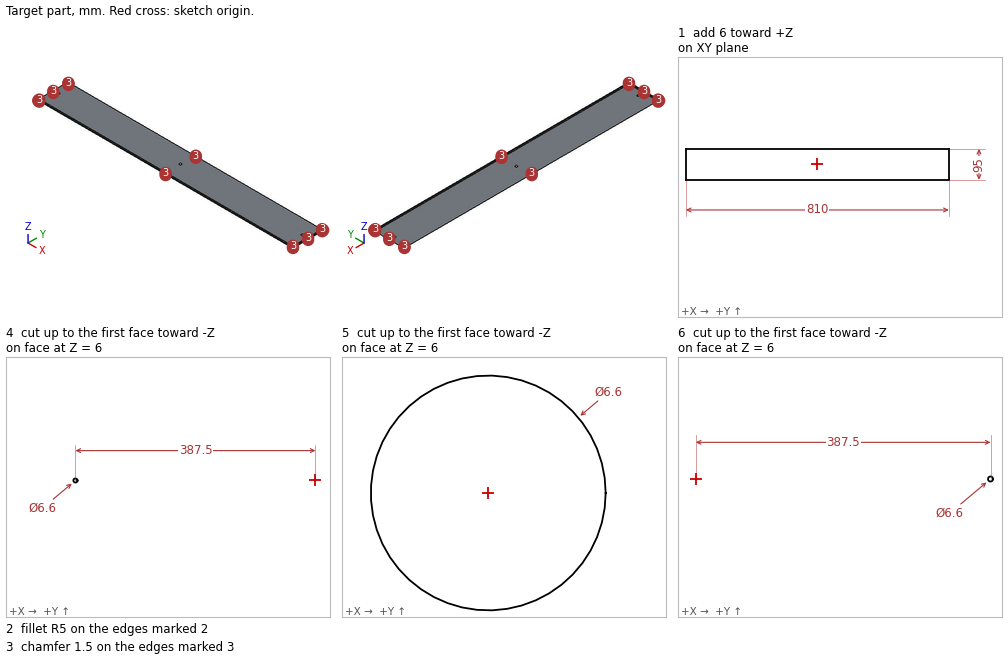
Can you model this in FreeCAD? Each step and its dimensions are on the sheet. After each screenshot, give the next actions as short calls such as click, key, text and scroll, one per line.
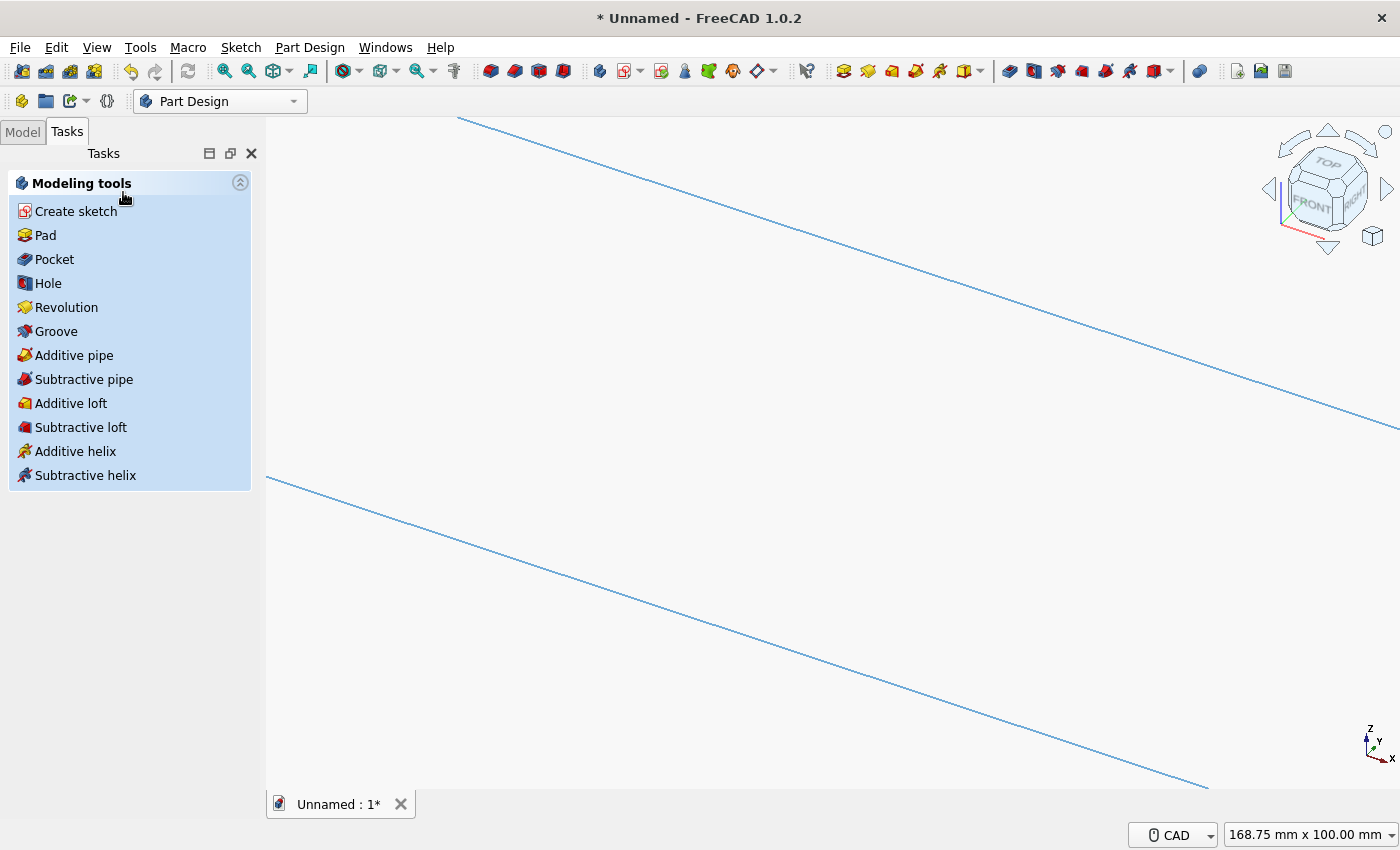
click(844, 72)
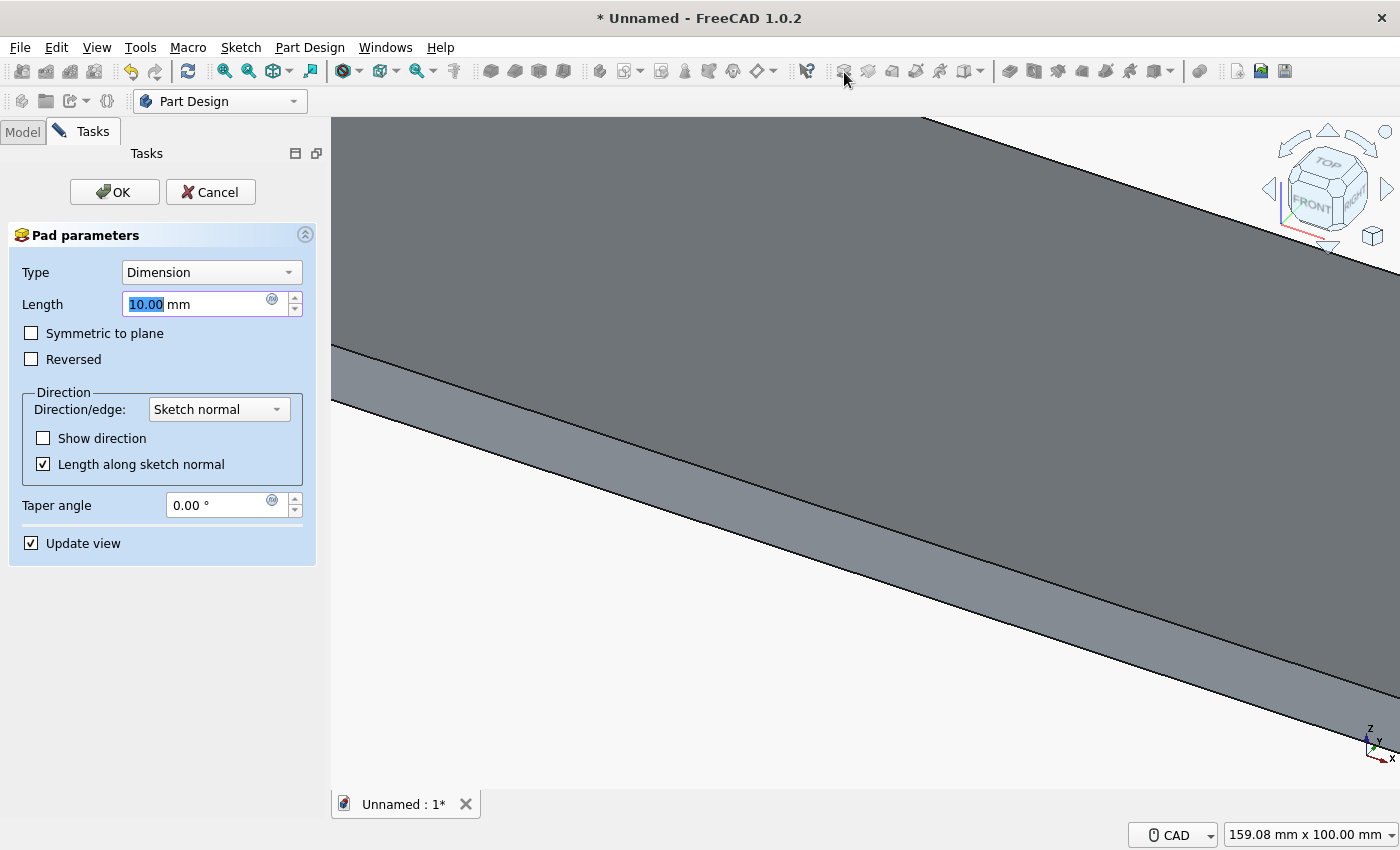
text(6)
key(Tab)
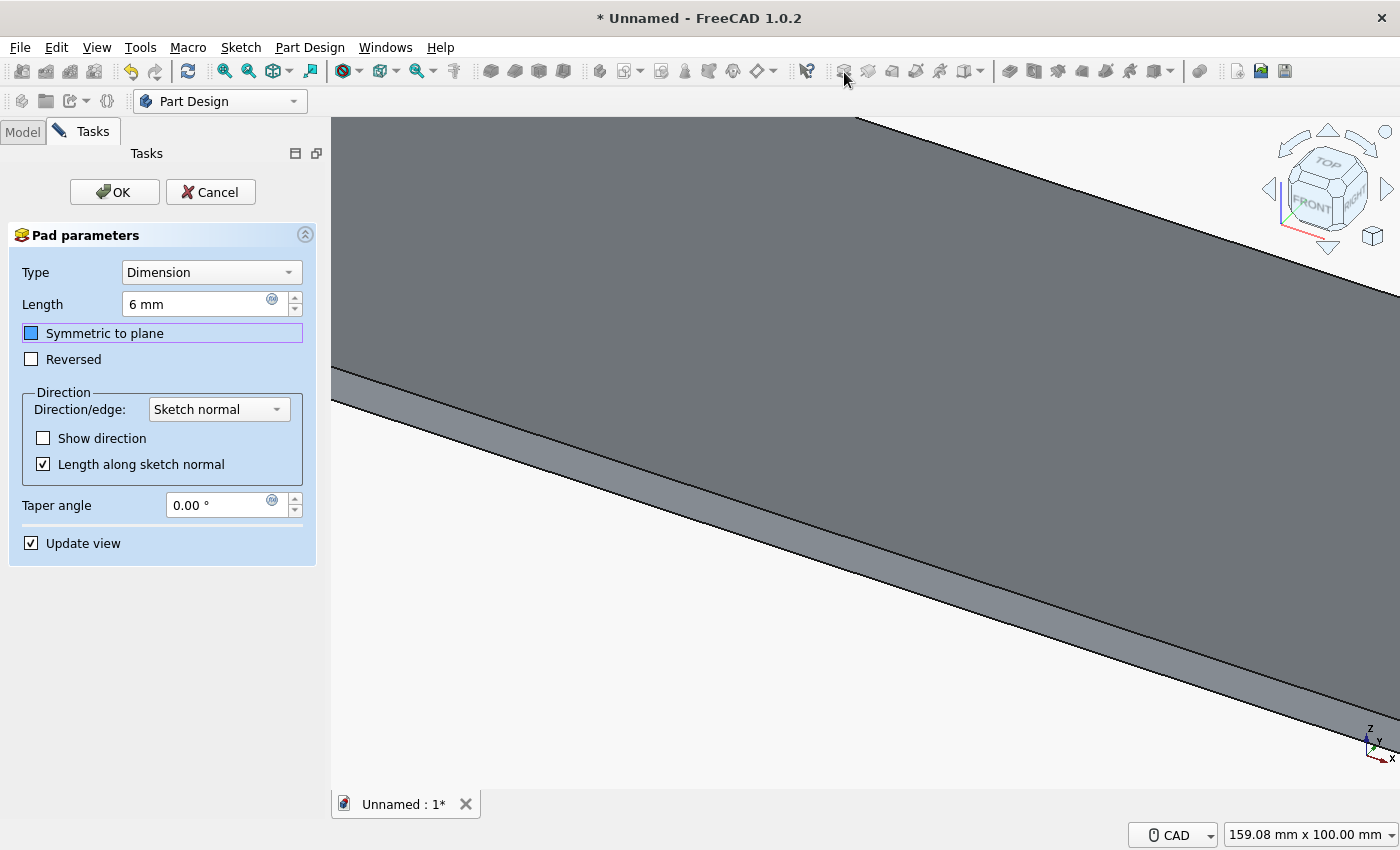
click(115, 192)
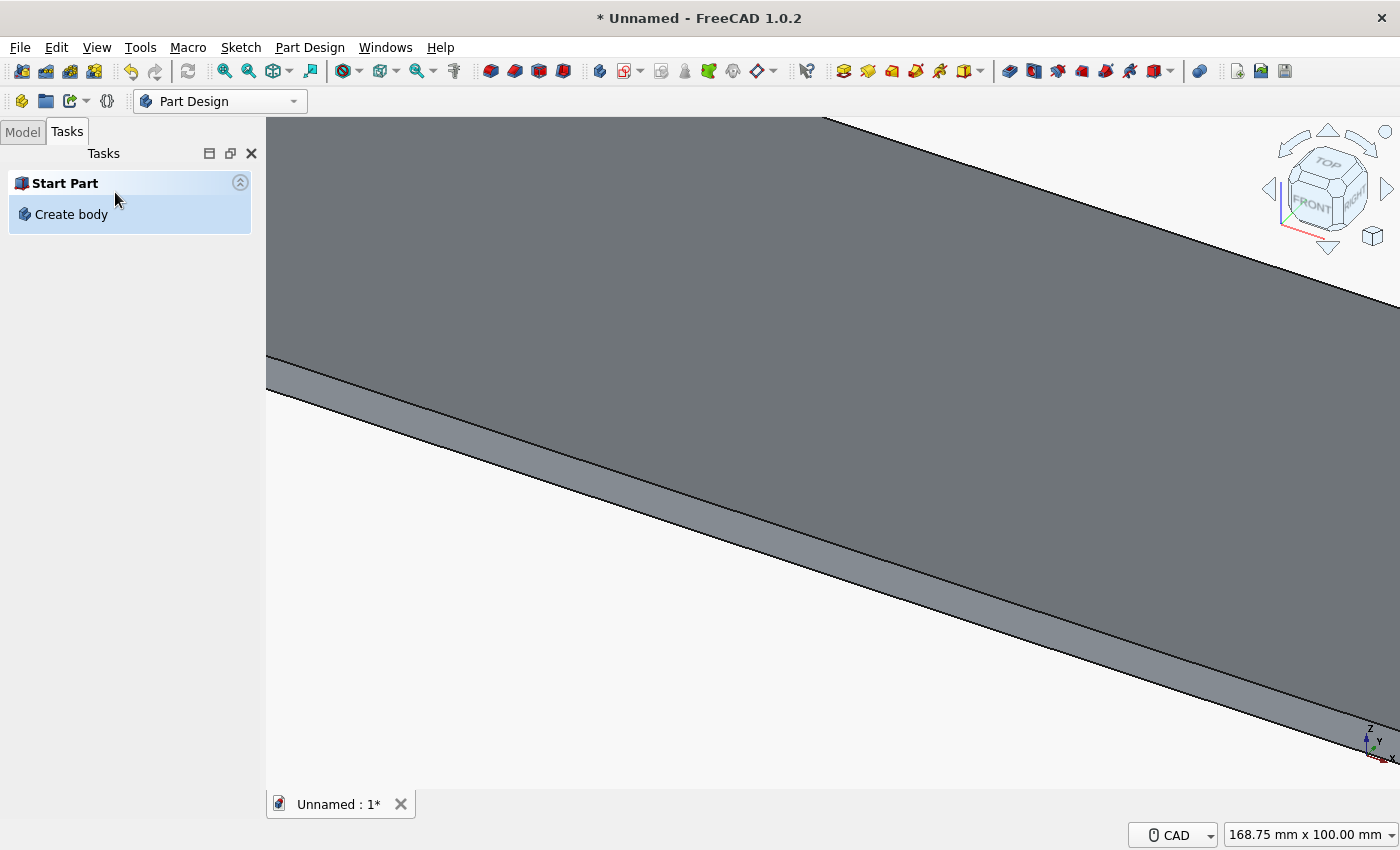
key(v)
key(f)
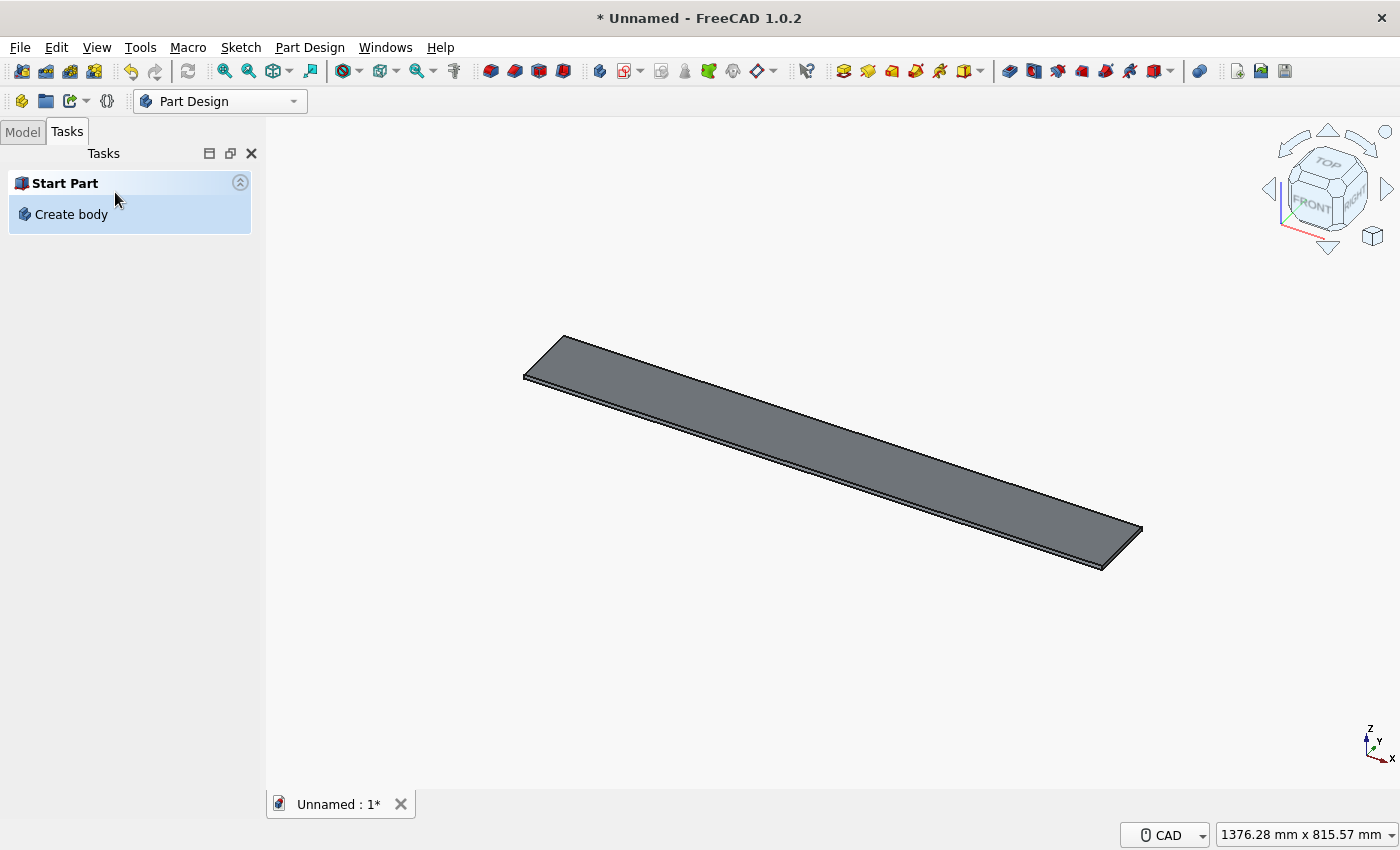
scroll(564, 337, up, 11)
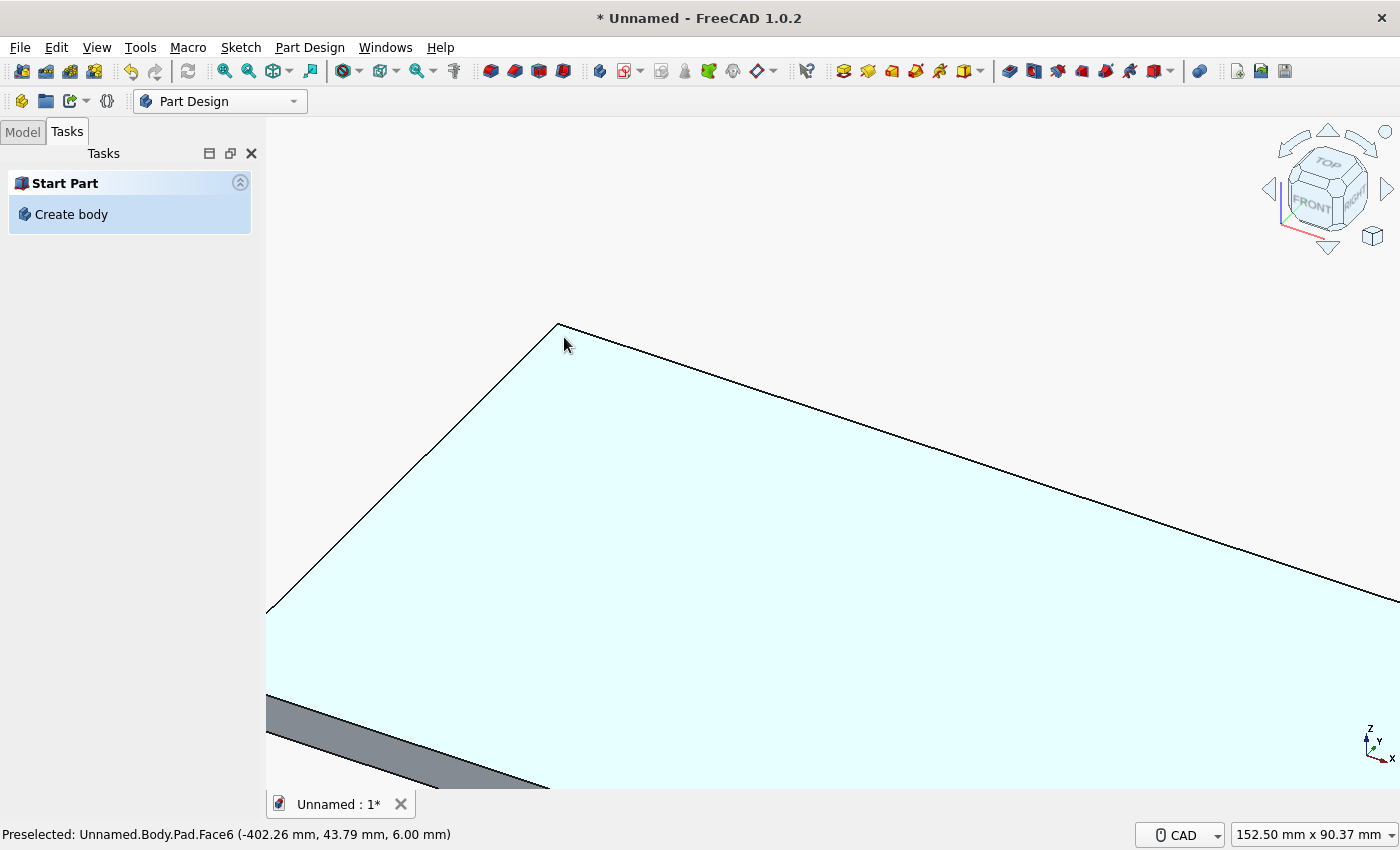
key(v)
key(f)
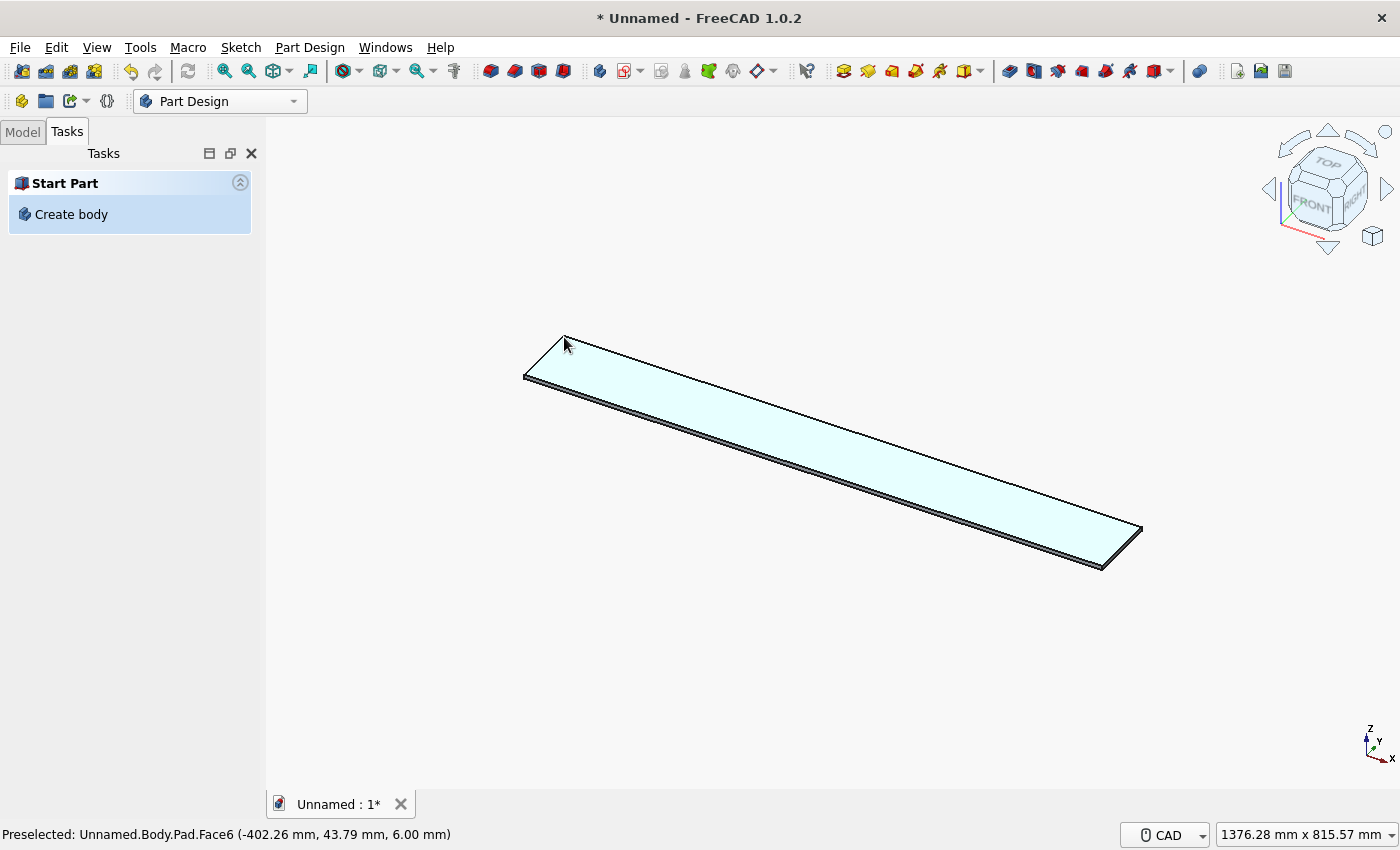
key(0)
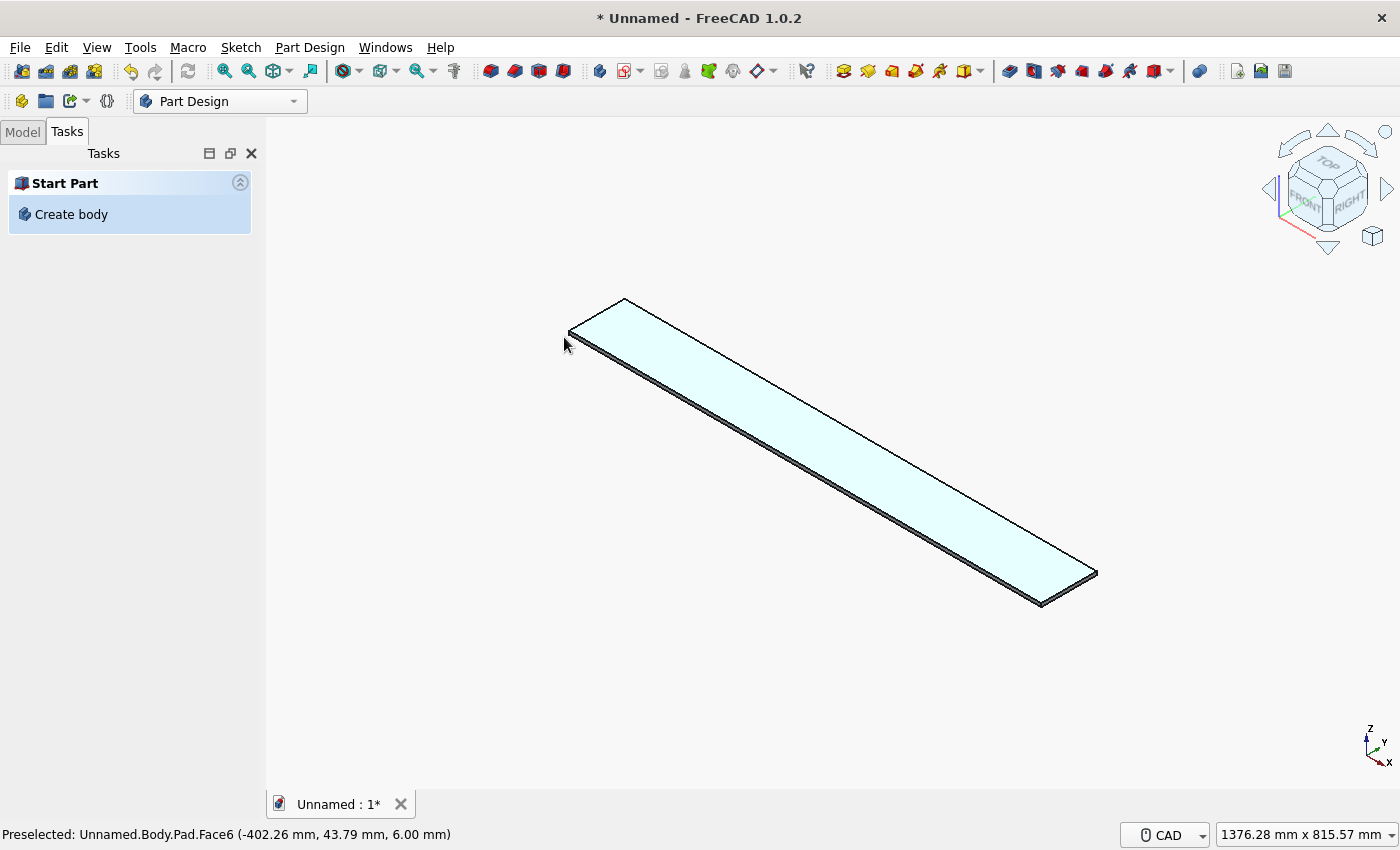
scroll(625, 300, up, 11)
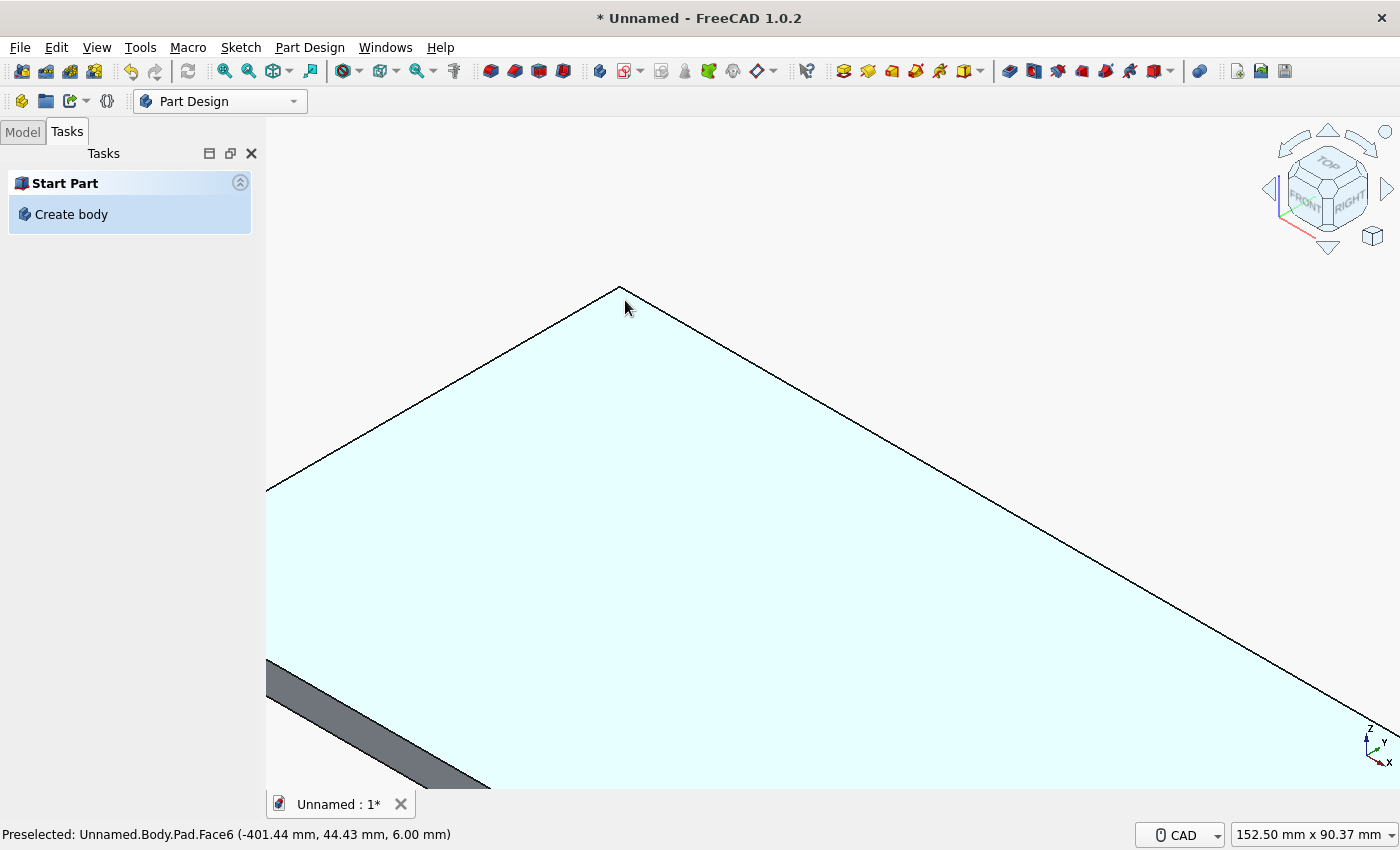
key(v)
key(f)